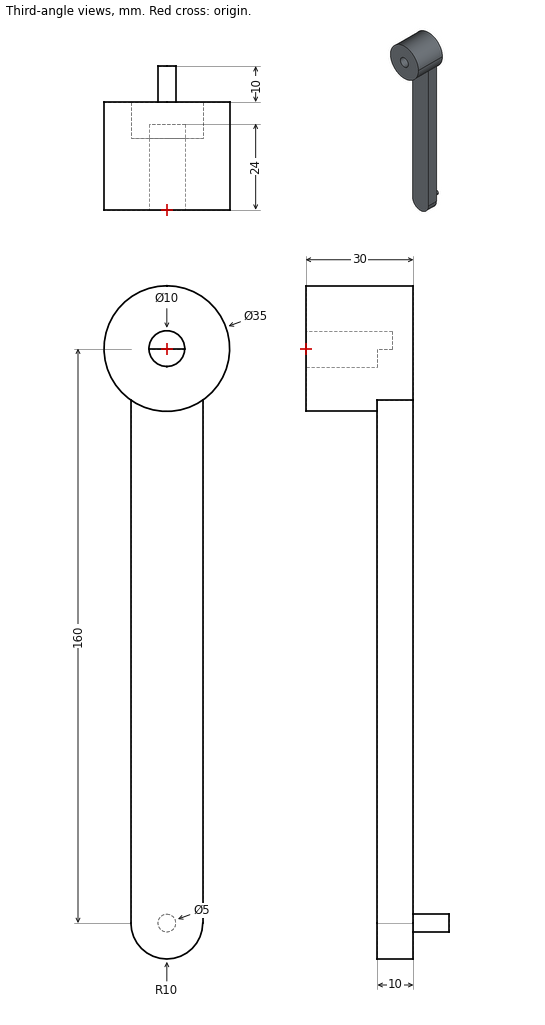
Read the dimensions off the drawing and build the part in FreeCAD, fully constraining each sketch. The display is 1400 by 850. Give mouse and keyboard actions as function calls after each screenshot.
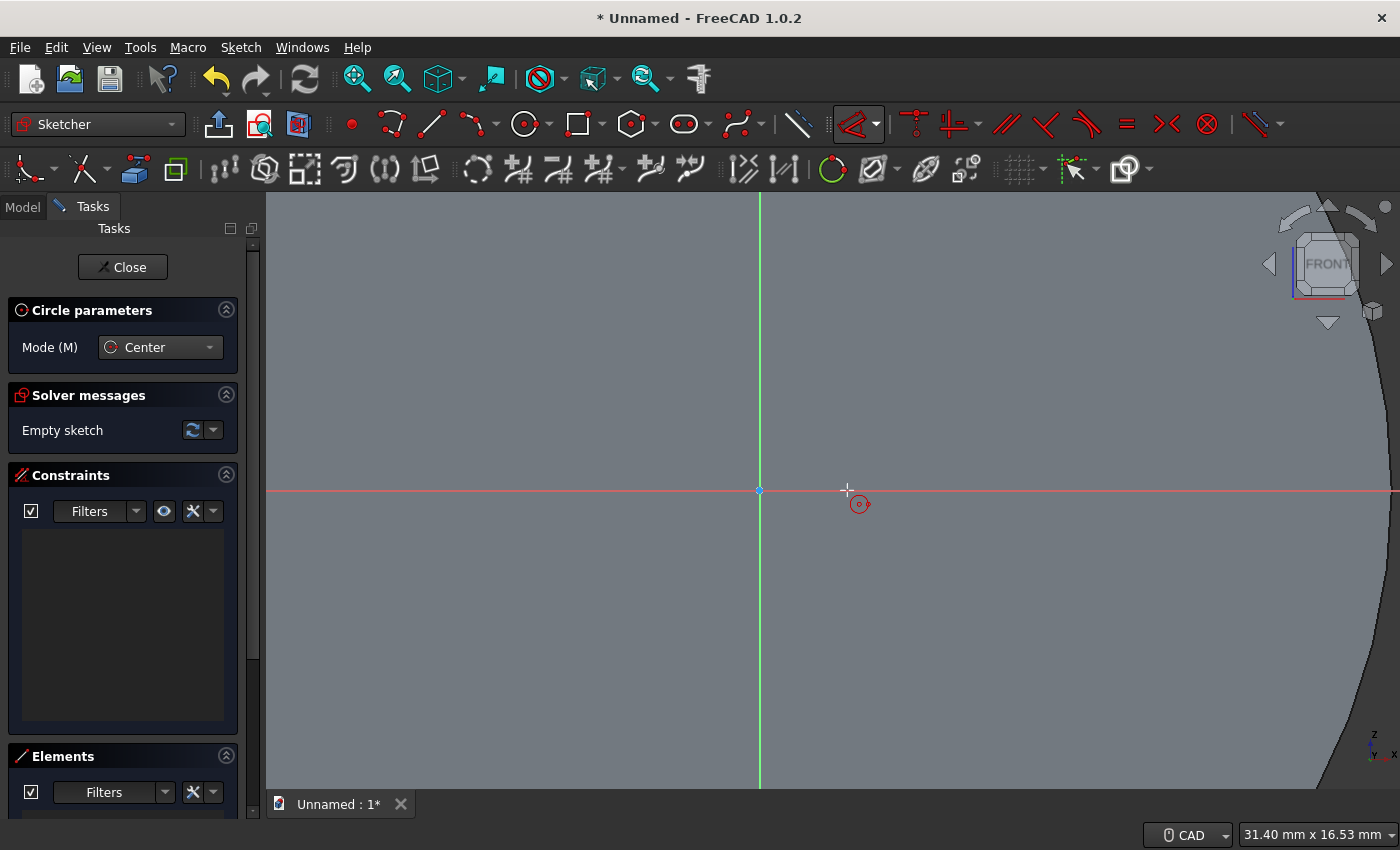
click(760, 490)
move(887, 363)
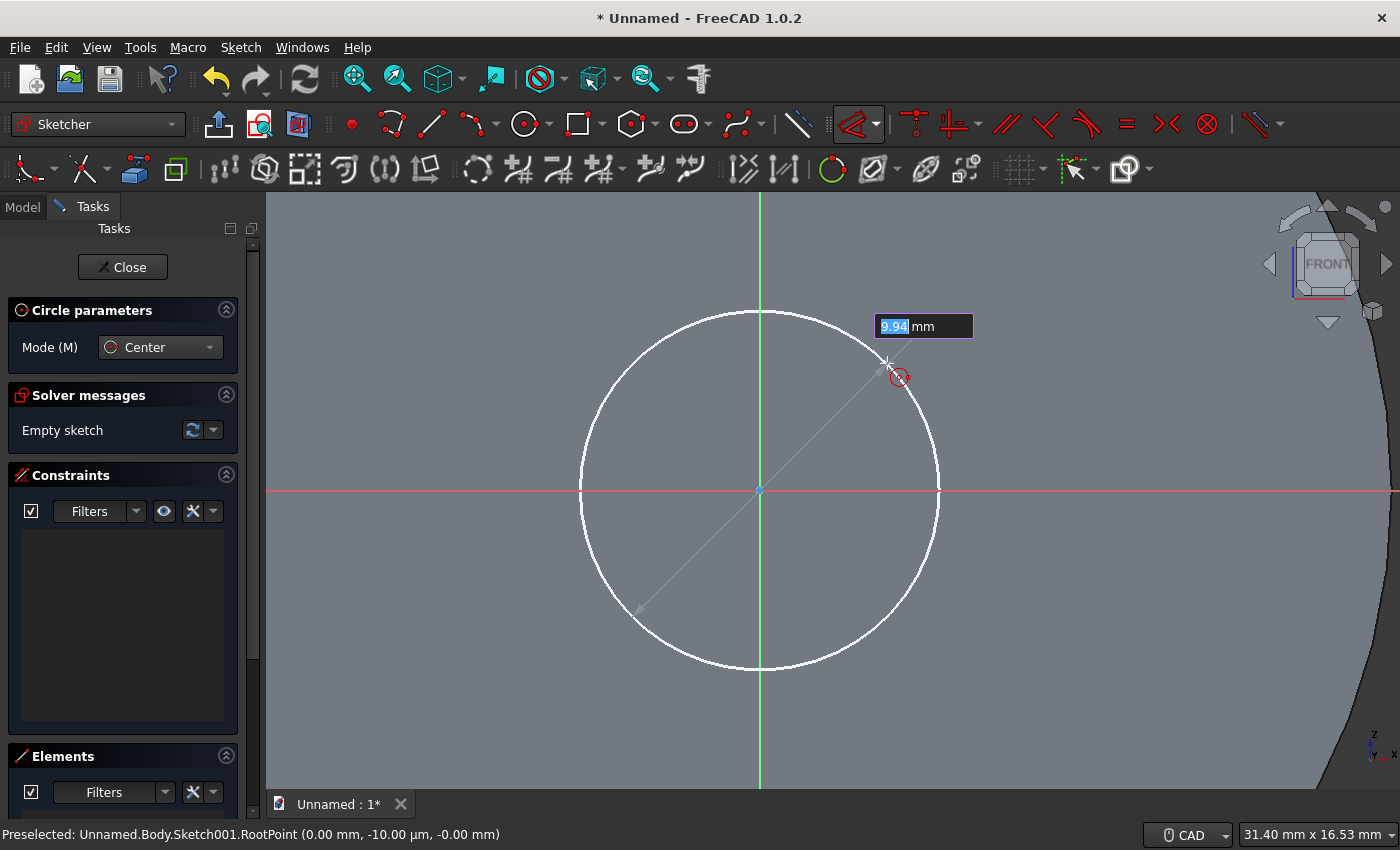
text(10)
key(Return)
key(Escape)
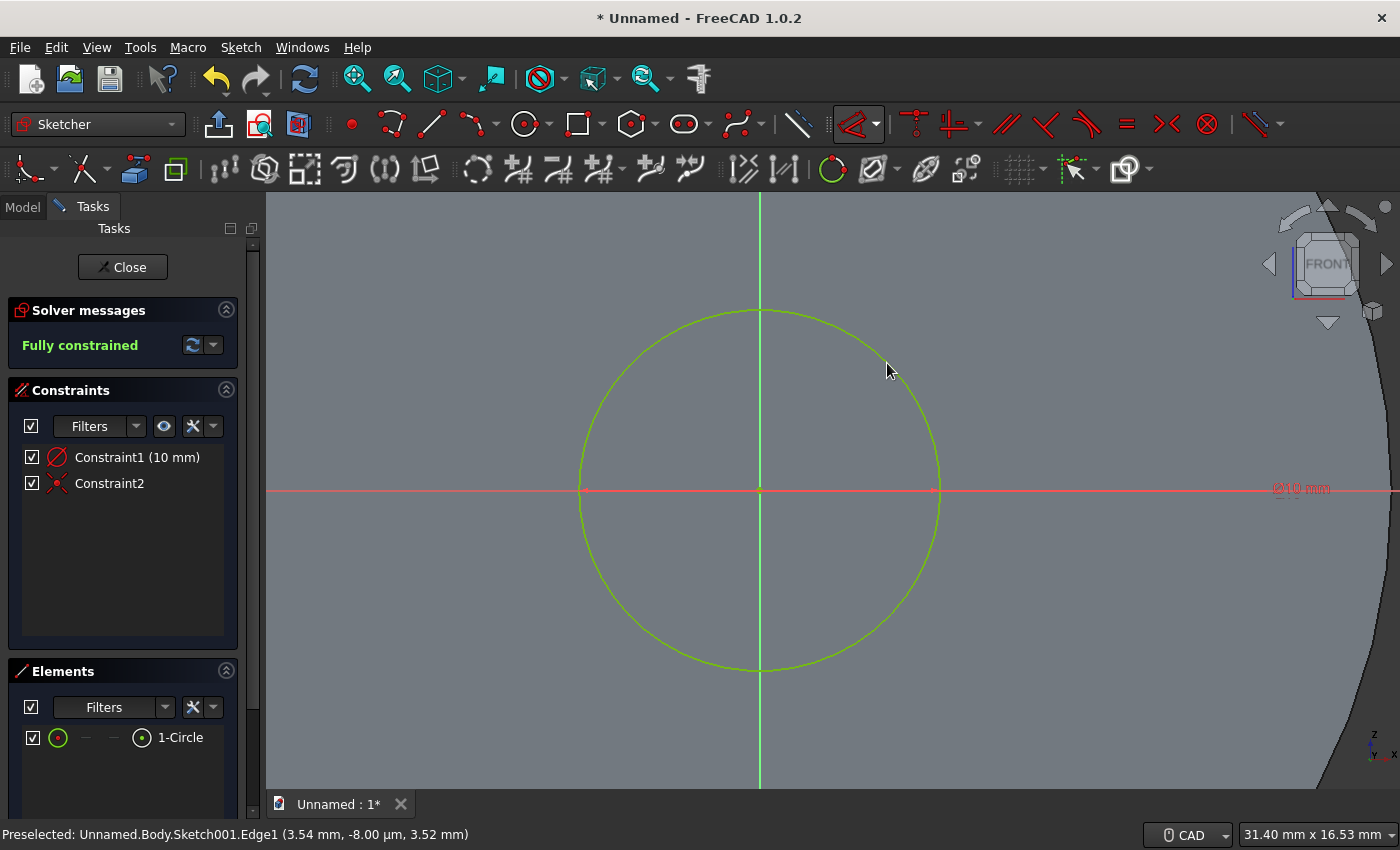
click(123, 267)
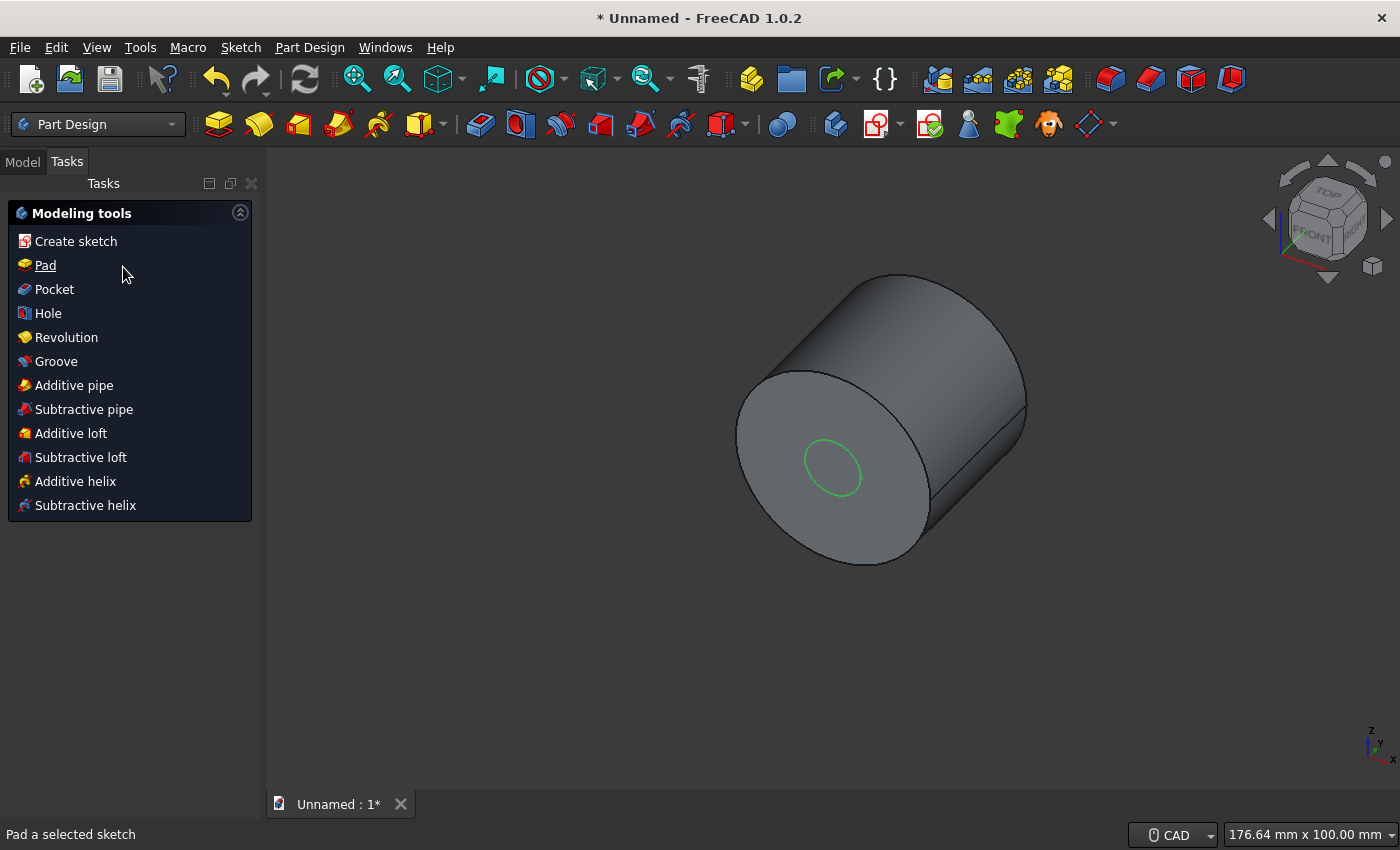
click(482, 124)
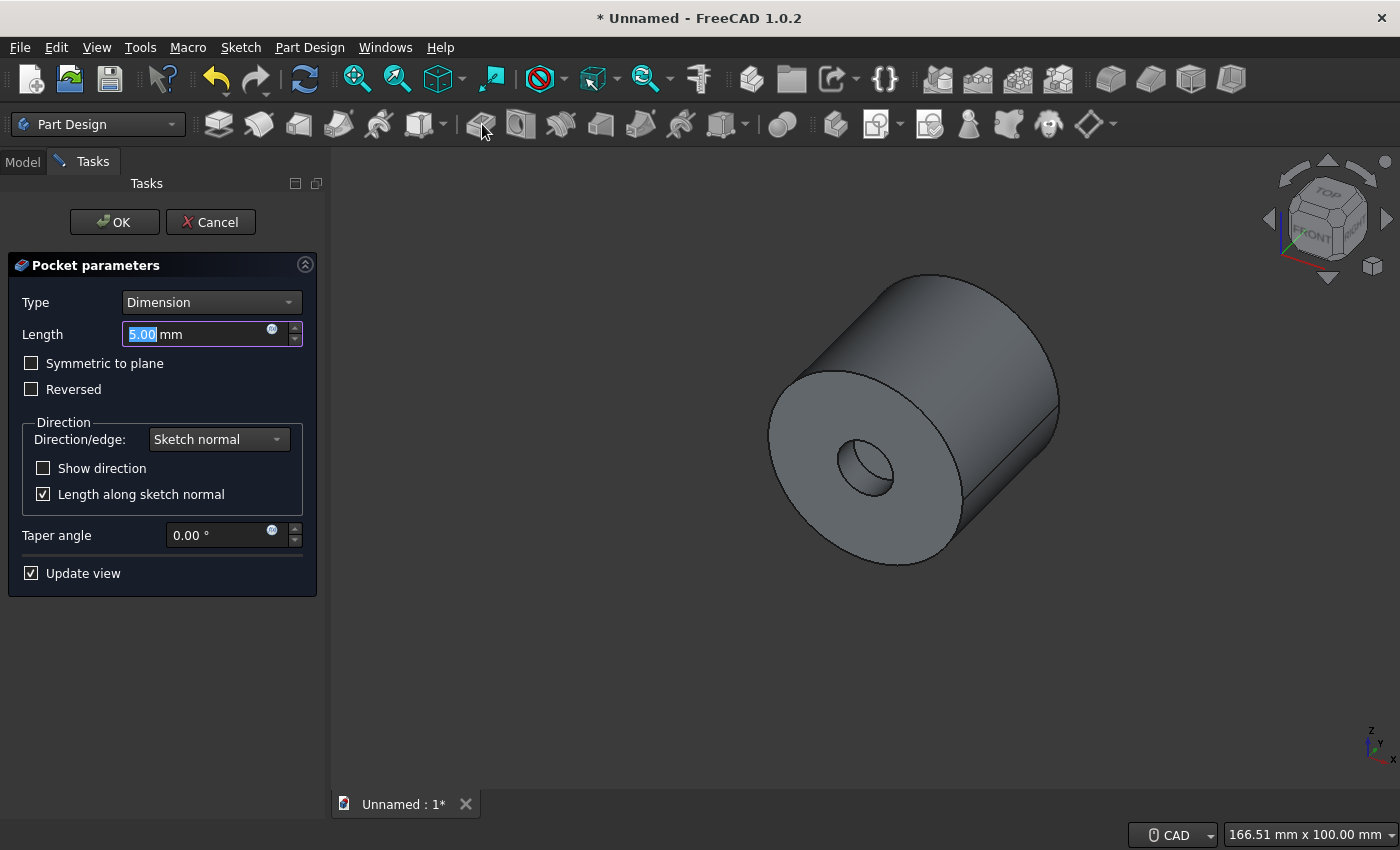
text(24)
key(Tab)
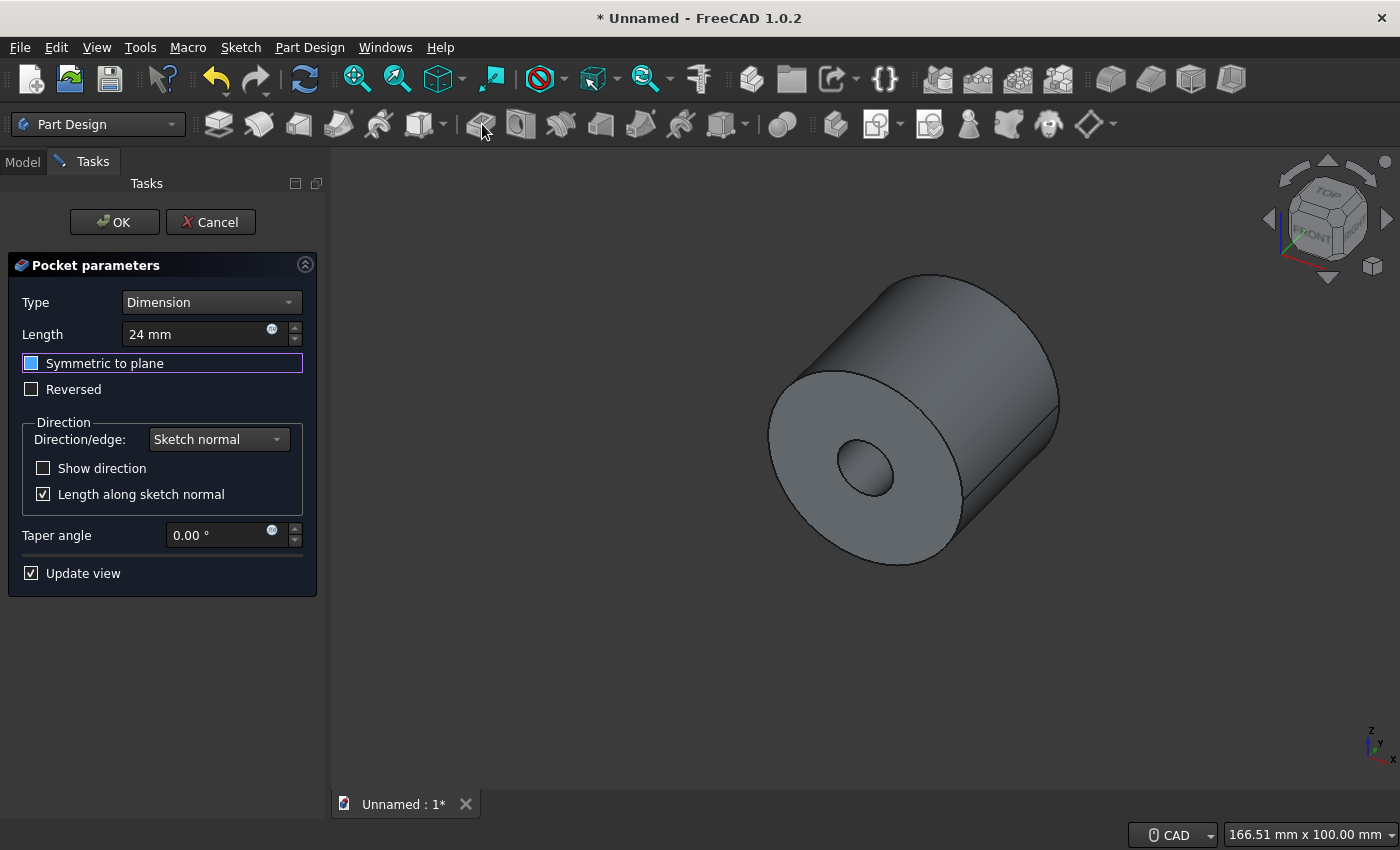
click(115, 222)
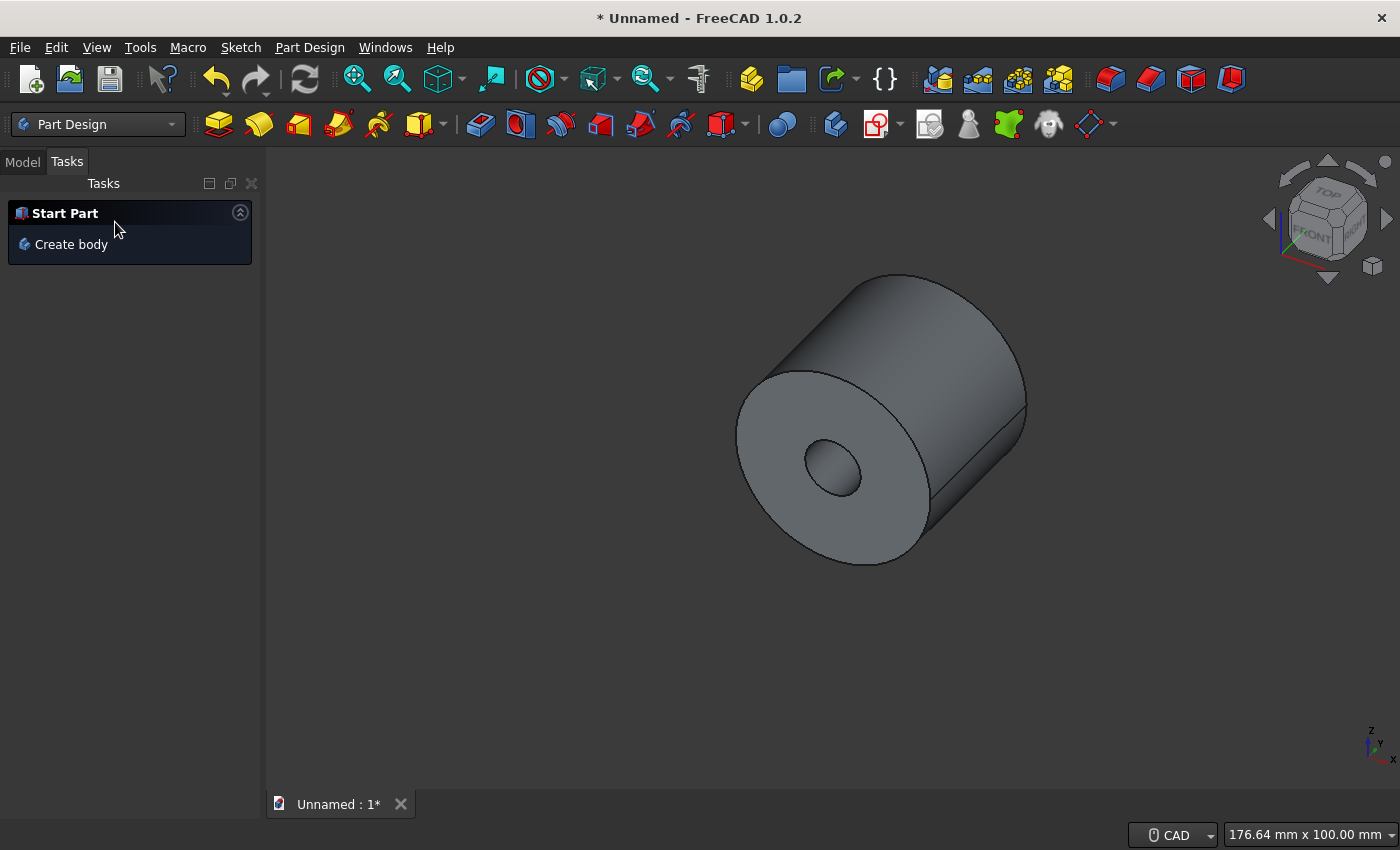
key(4)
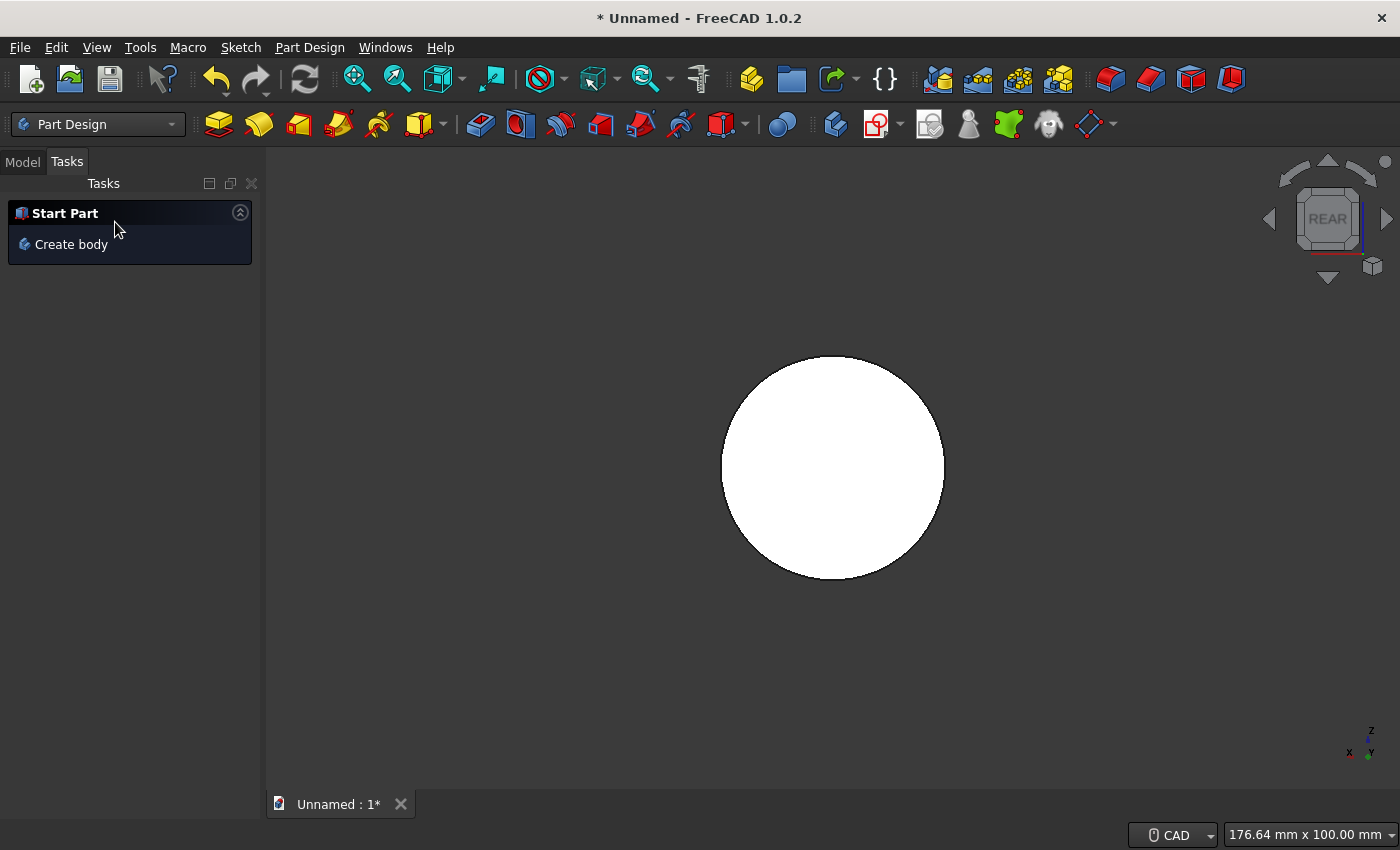
click(358, 80)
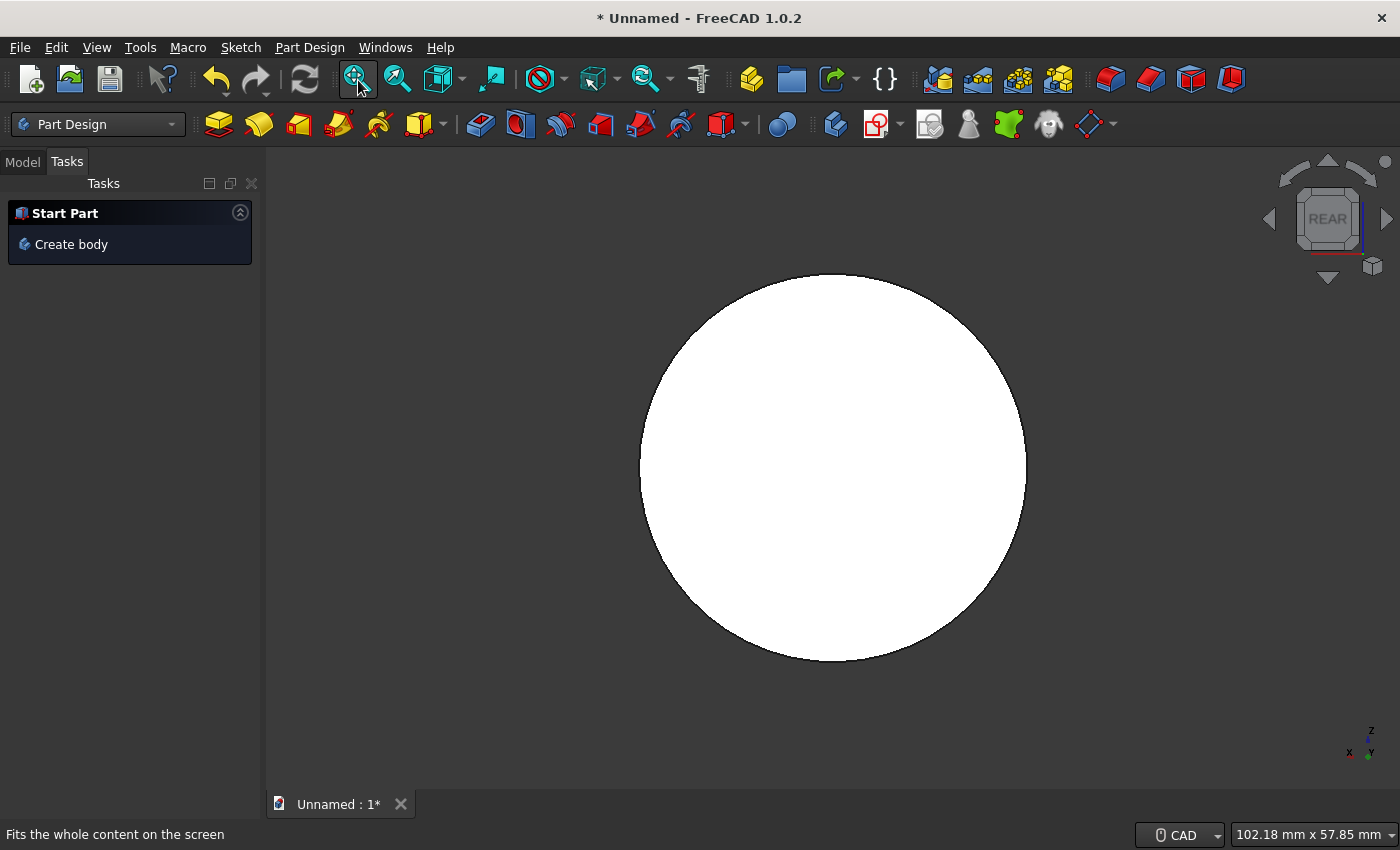
click(833, 467)